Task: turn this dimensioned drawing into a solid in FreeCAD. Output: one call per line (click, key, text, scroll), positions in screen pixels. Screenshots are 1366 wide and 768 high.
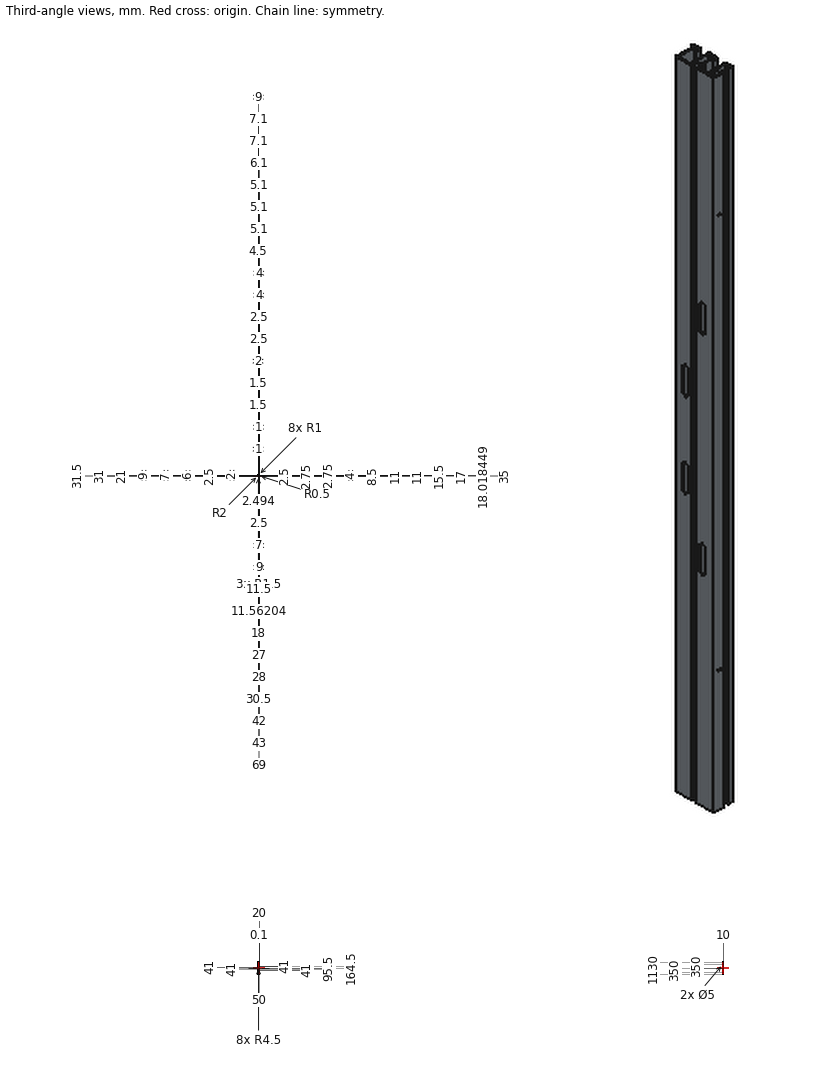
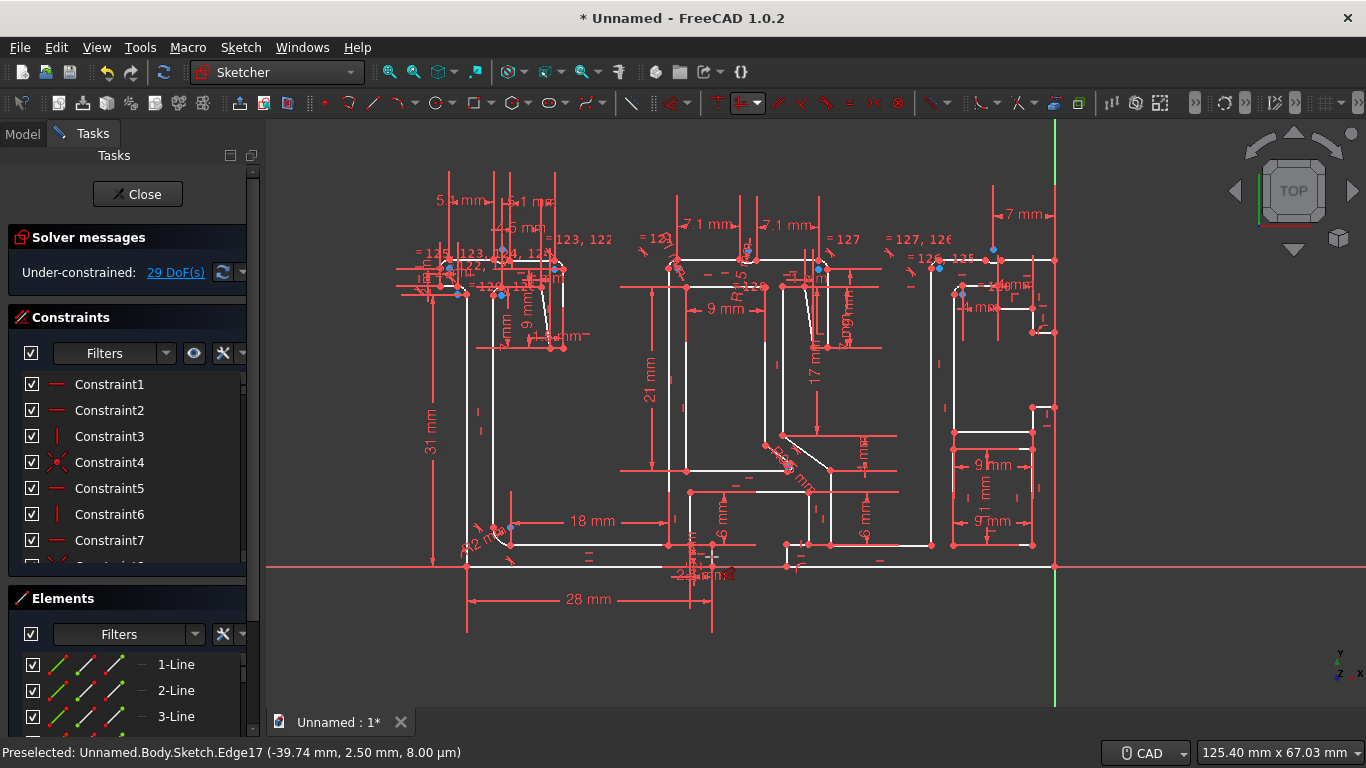
scroll(1048, 407, up, 4)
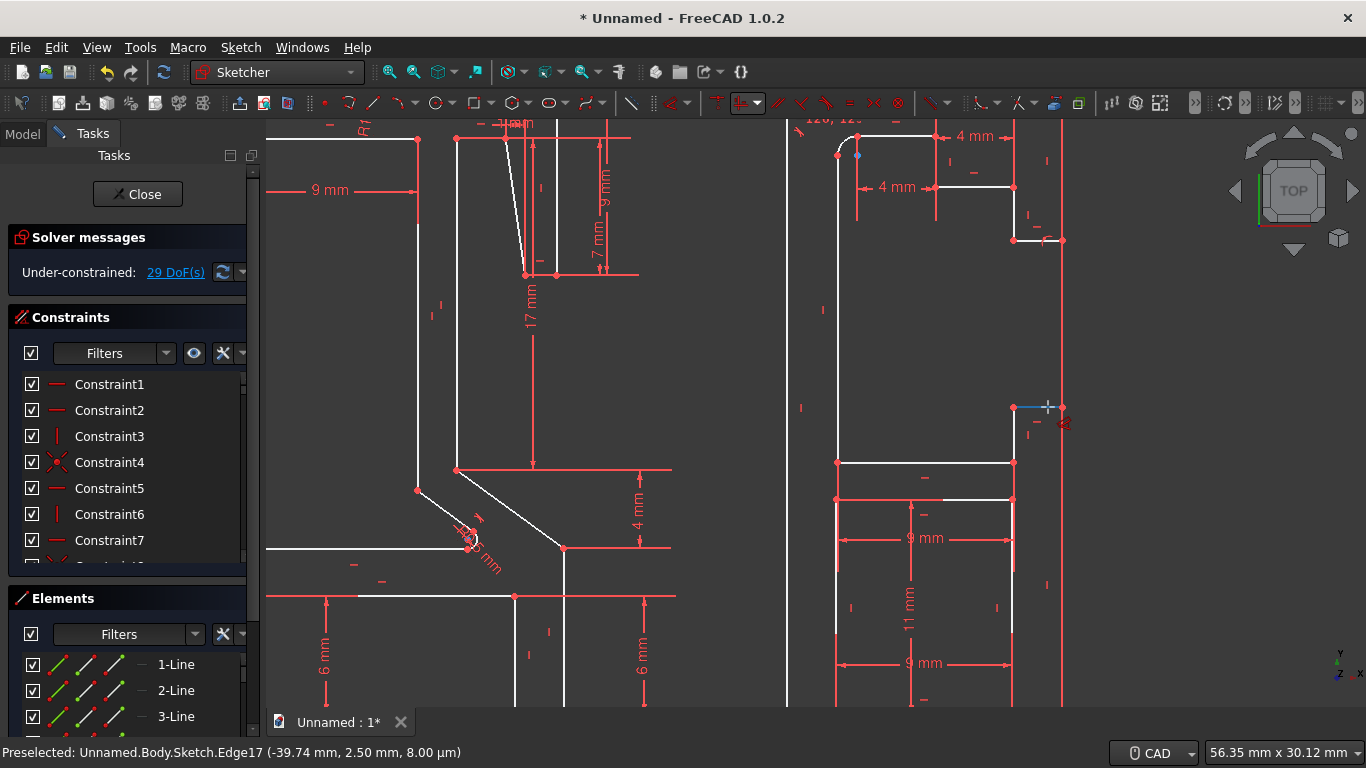
click(1048, 407)
click(1038, 373)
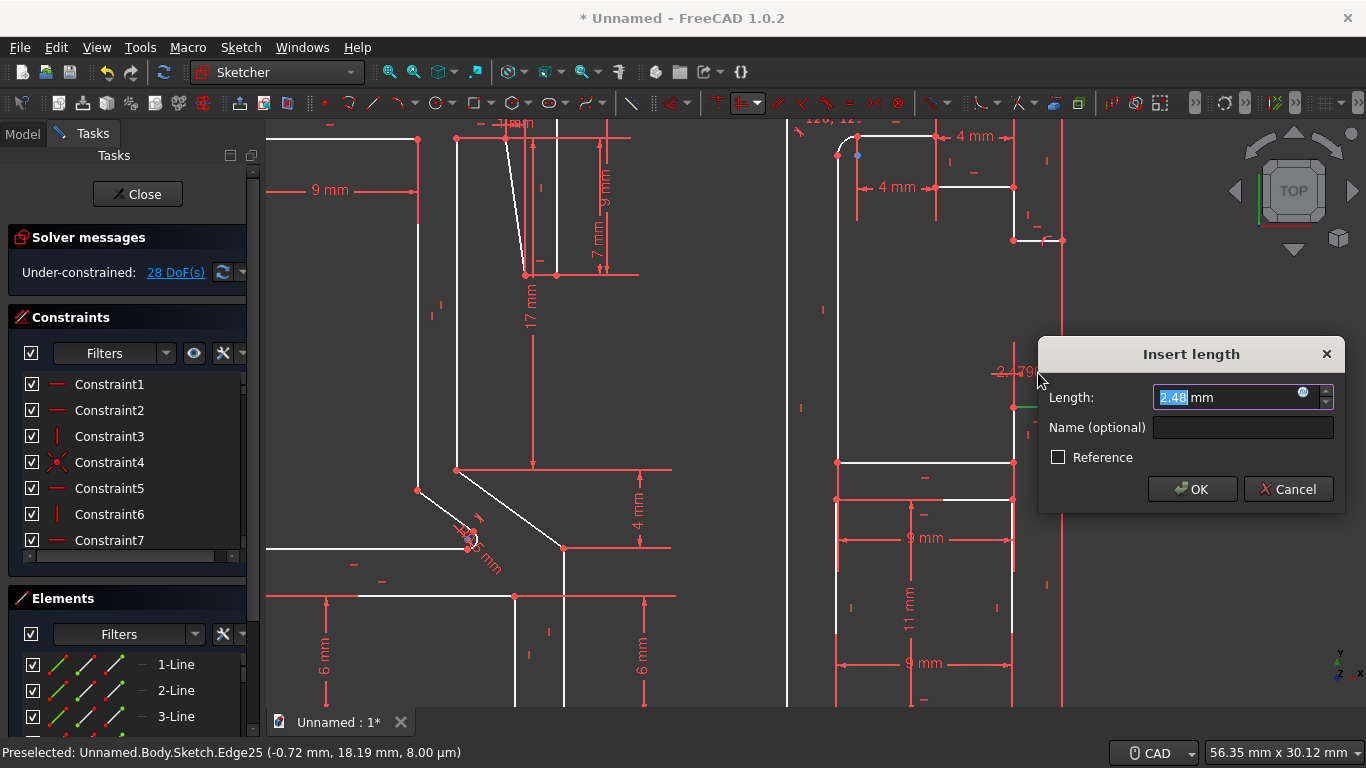
text(2.5)
key(Return)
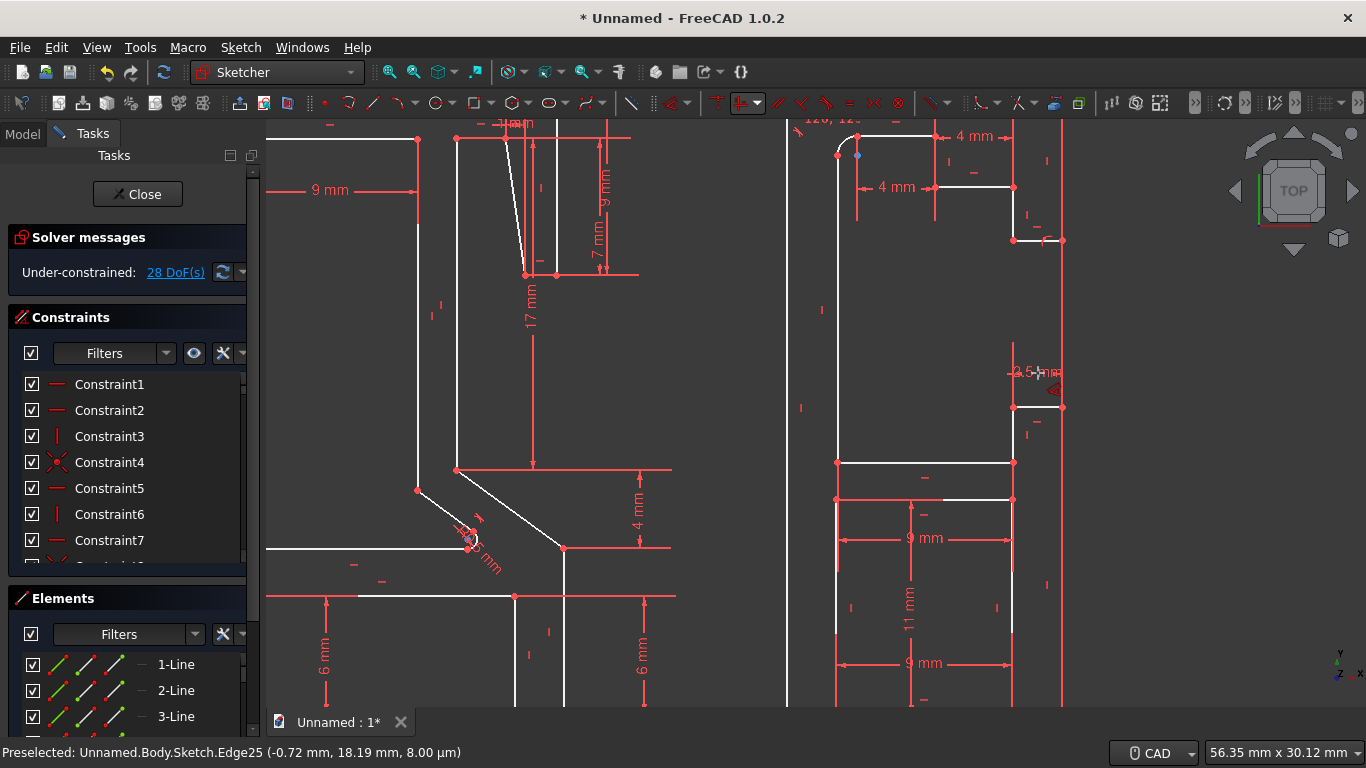
click(935, 152)
click(969, 167)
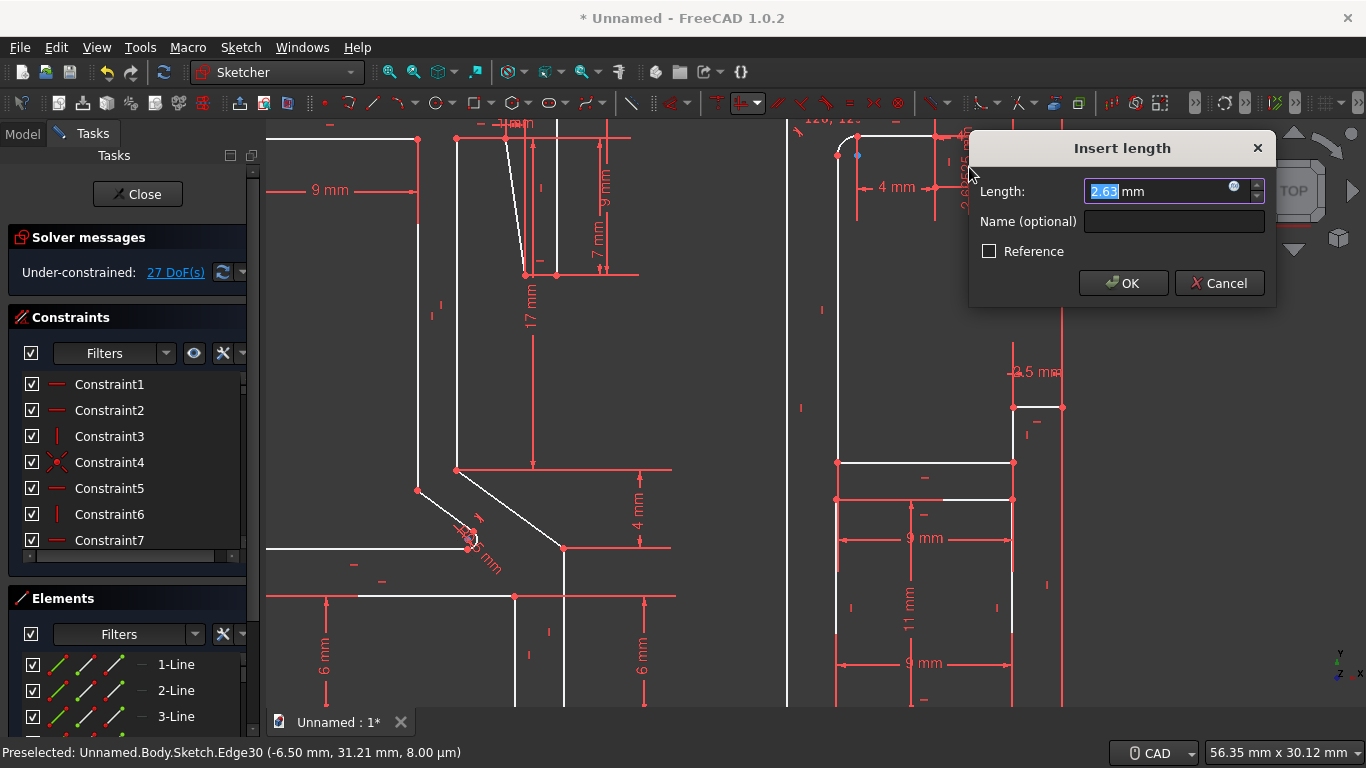
text(2.5)
key(Return)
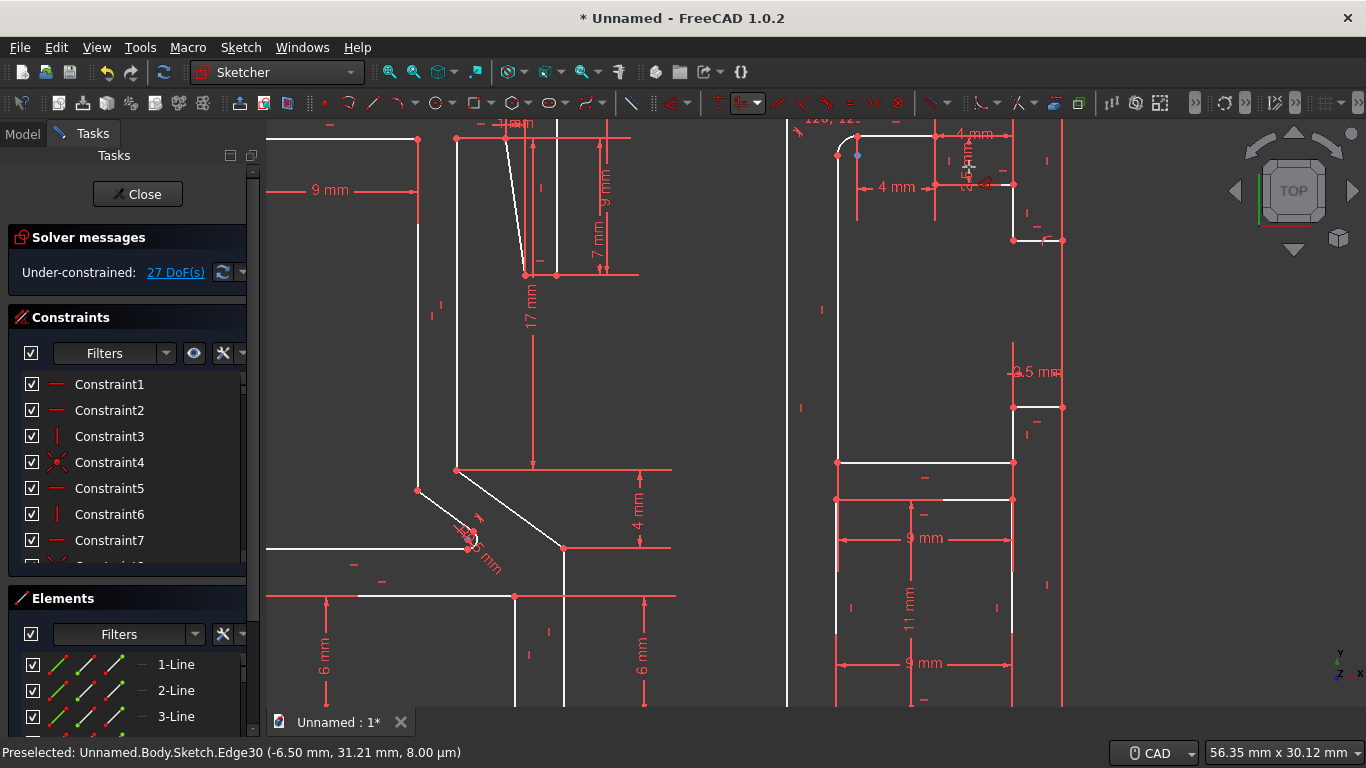
scroll(1048, 407, down, 4)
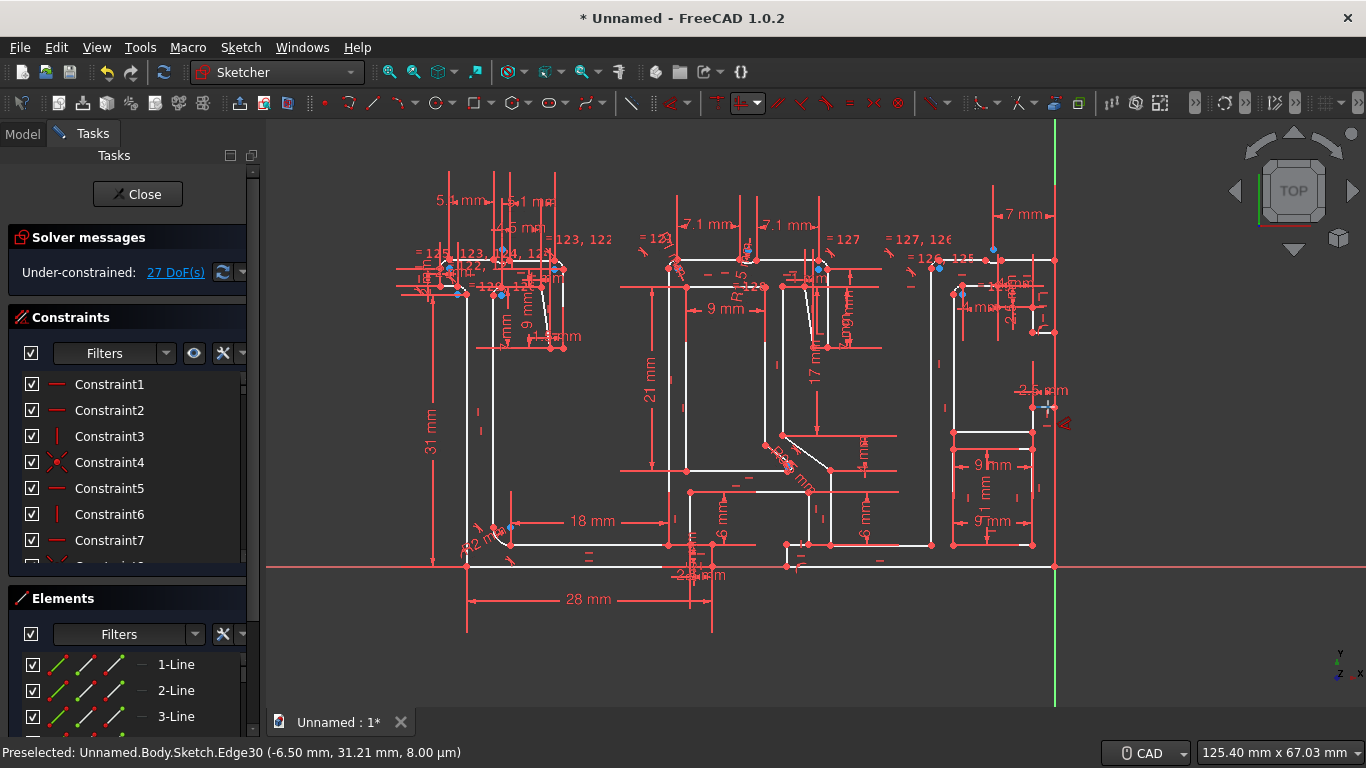
click(1039, 260)
click(1028, 178)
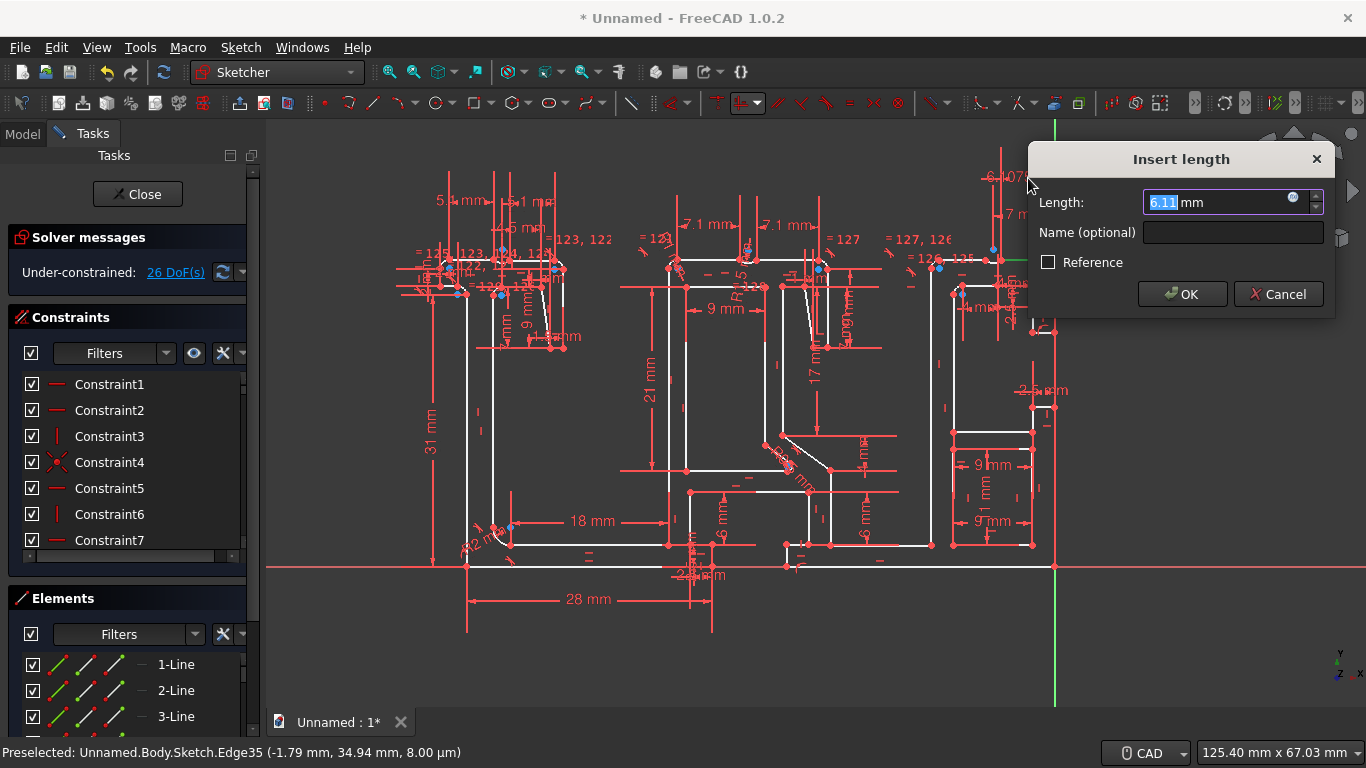
text(6.1)
key(Return)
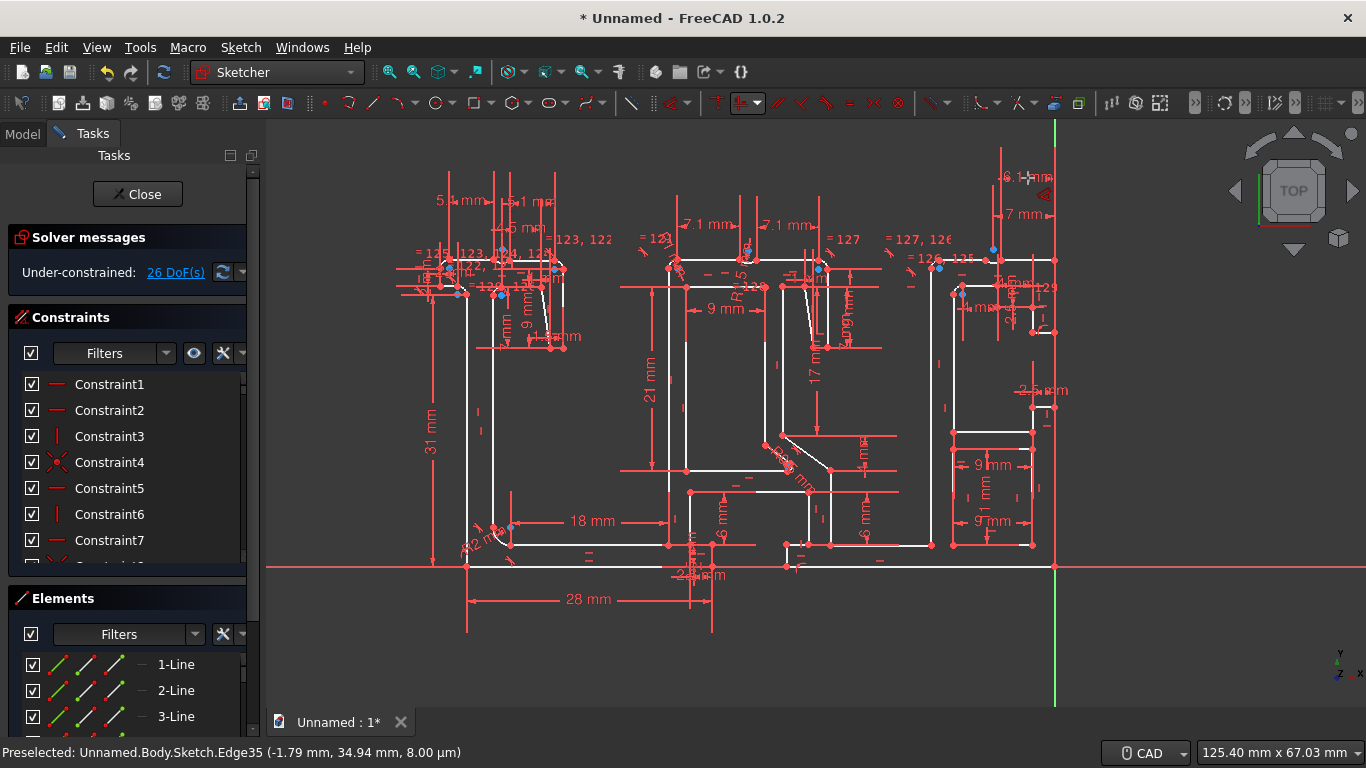
click(972, 260)
click(952, 226)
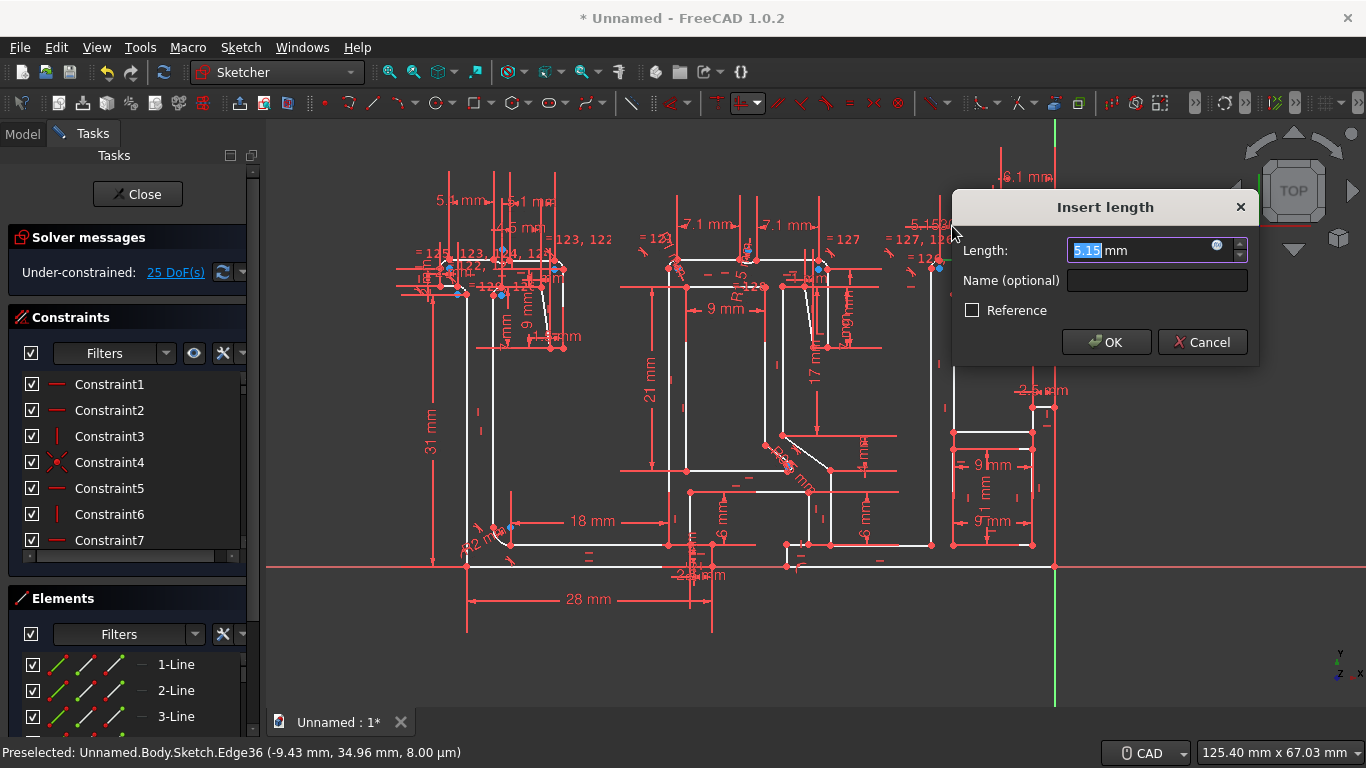
text(5.1)
key(Return)